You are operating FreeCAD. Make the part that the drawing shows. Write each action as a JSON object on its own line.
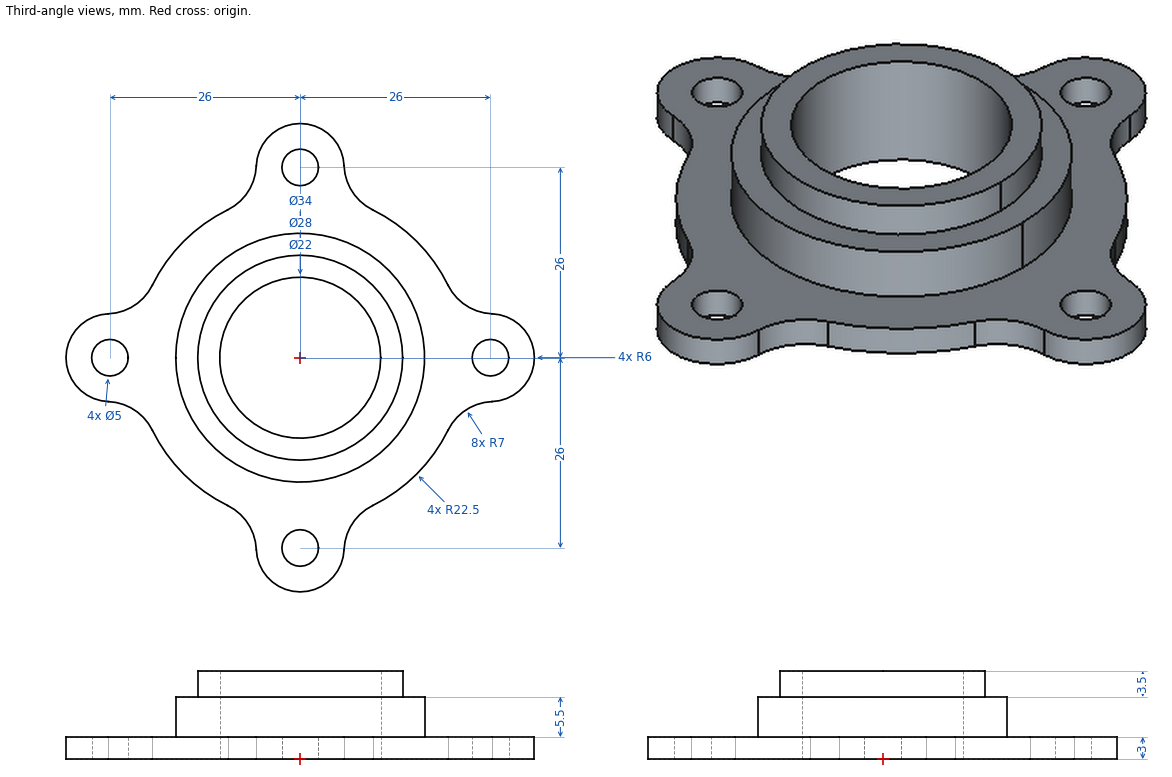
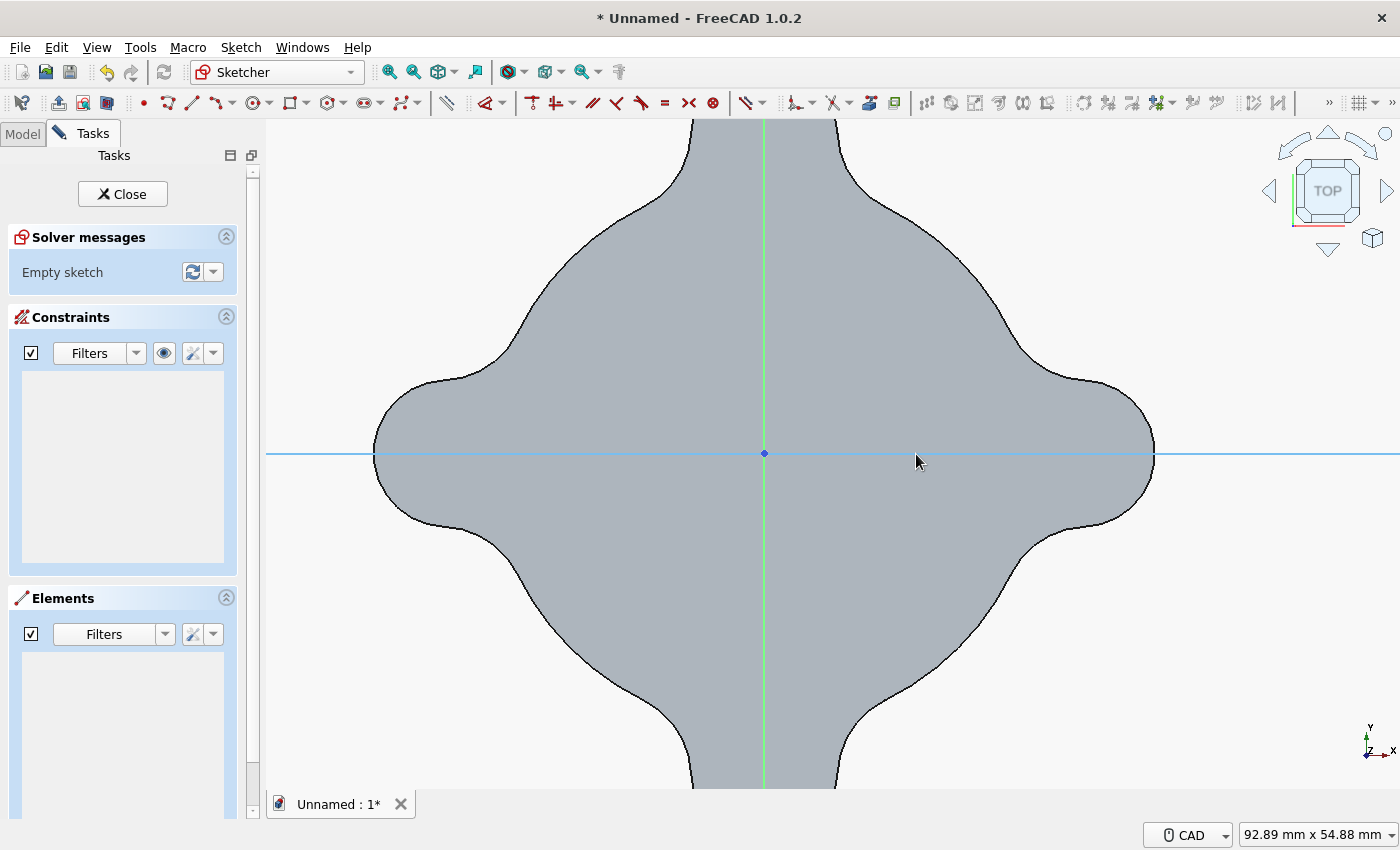
{"action": "left_click", "coordinate": [254, 104]}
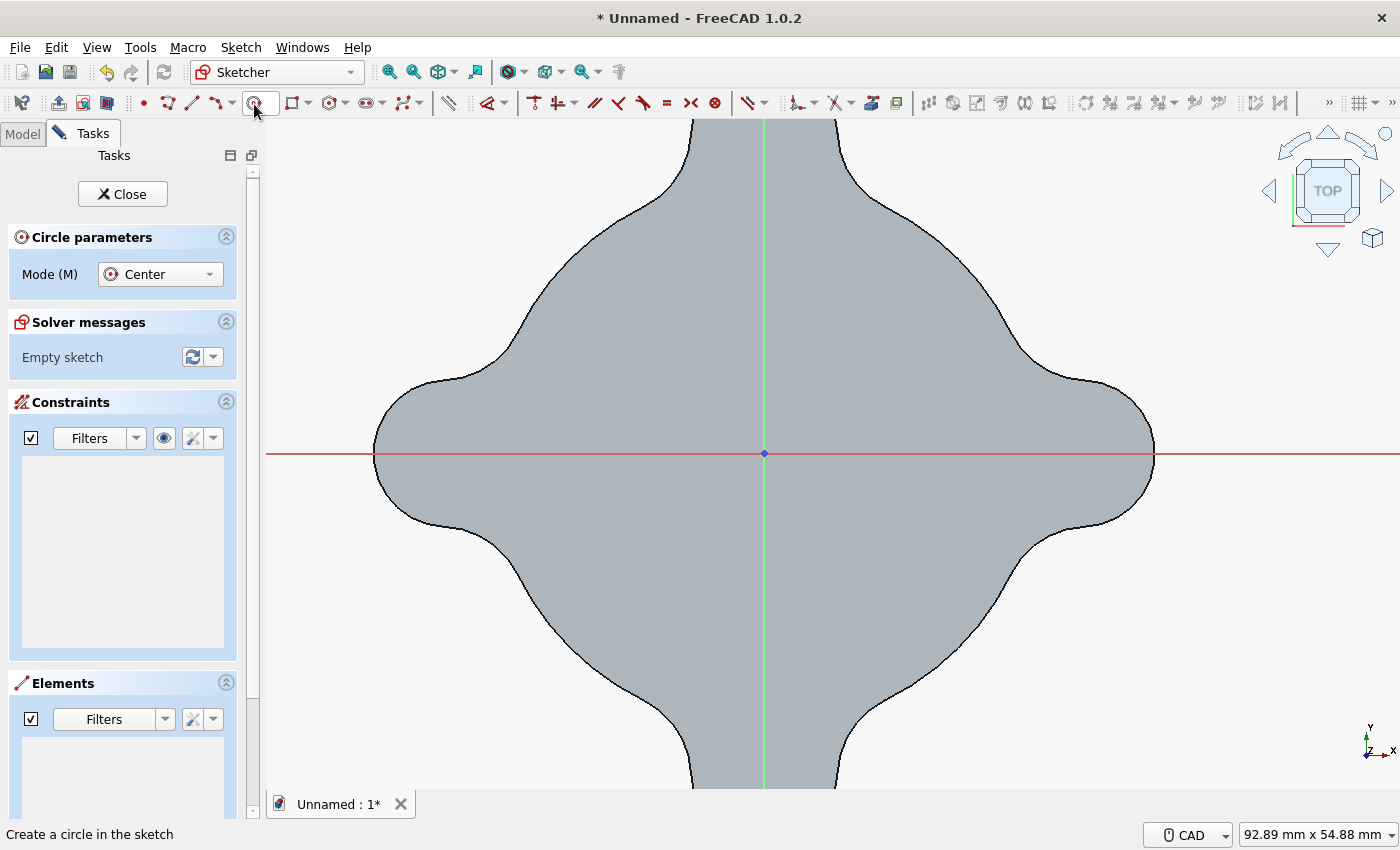
{"action": "left_click", "coordinate": [764, 454]}
{"action": "mouse_move", "coordinate": [911, 307]}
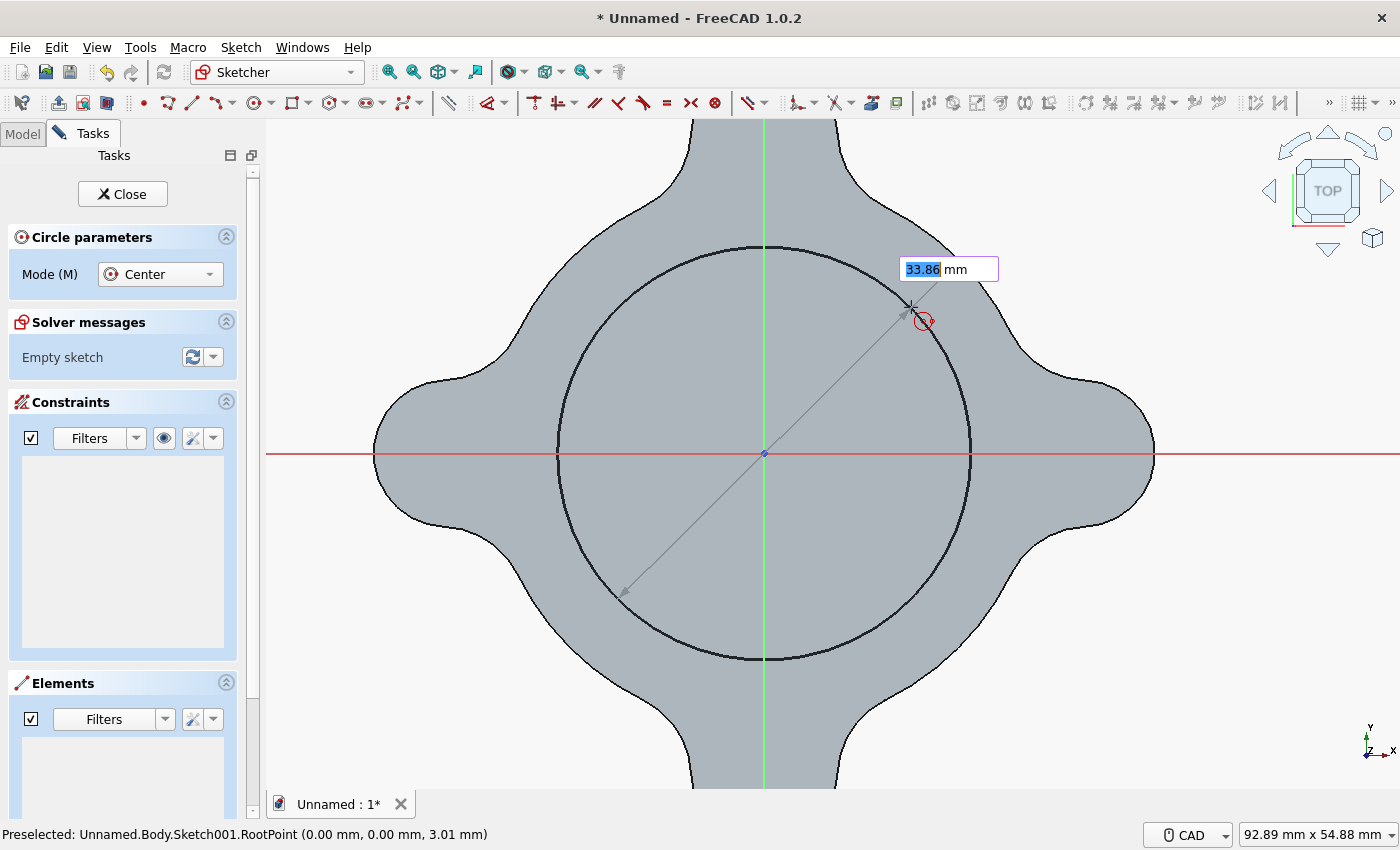
{"action": "type", "text": "34"}
{"action": "key", "text": "Return"}
{"action": "key", "text": "Escape"}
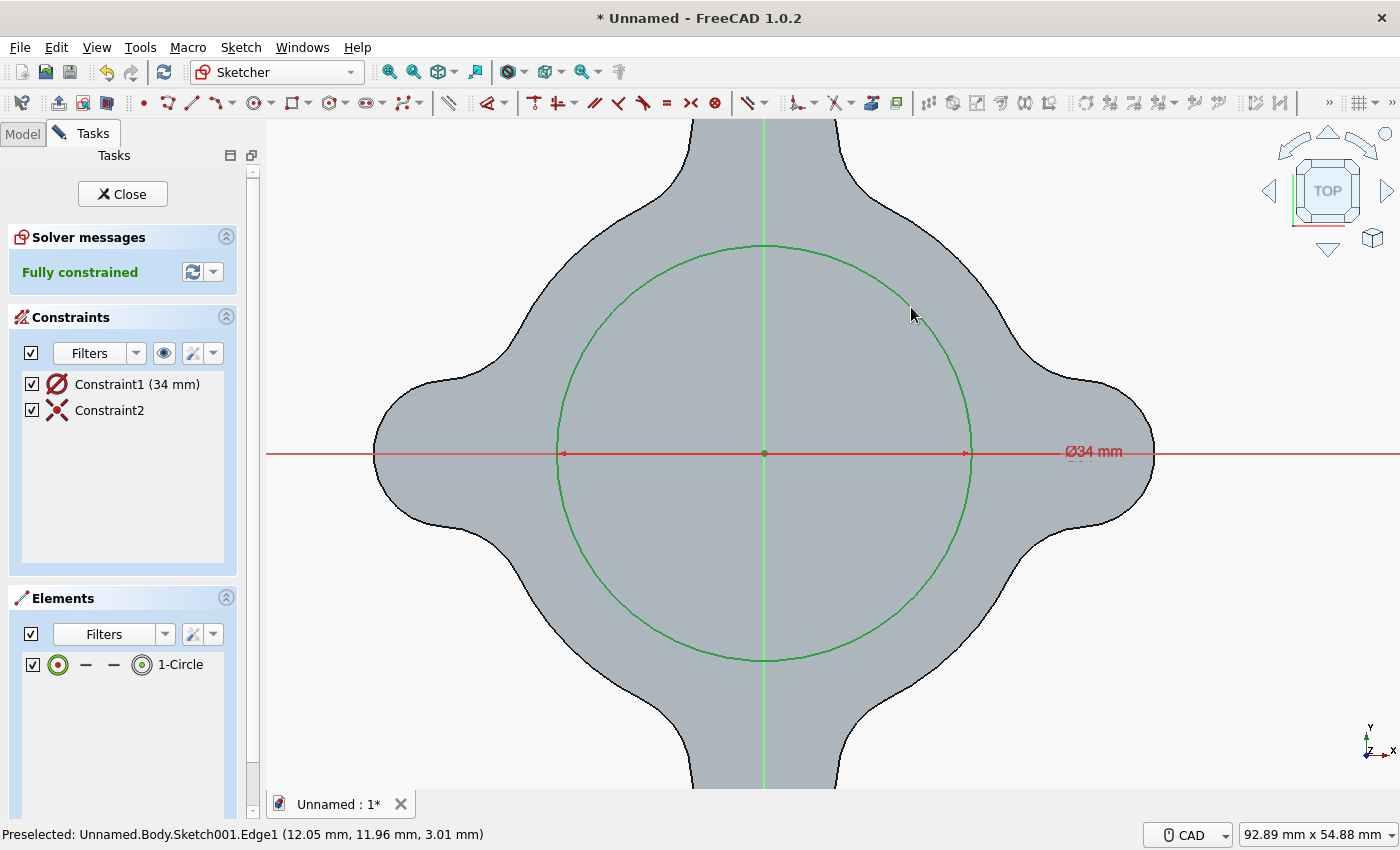
{"action": "left_click", "coordinate": [123, 194]}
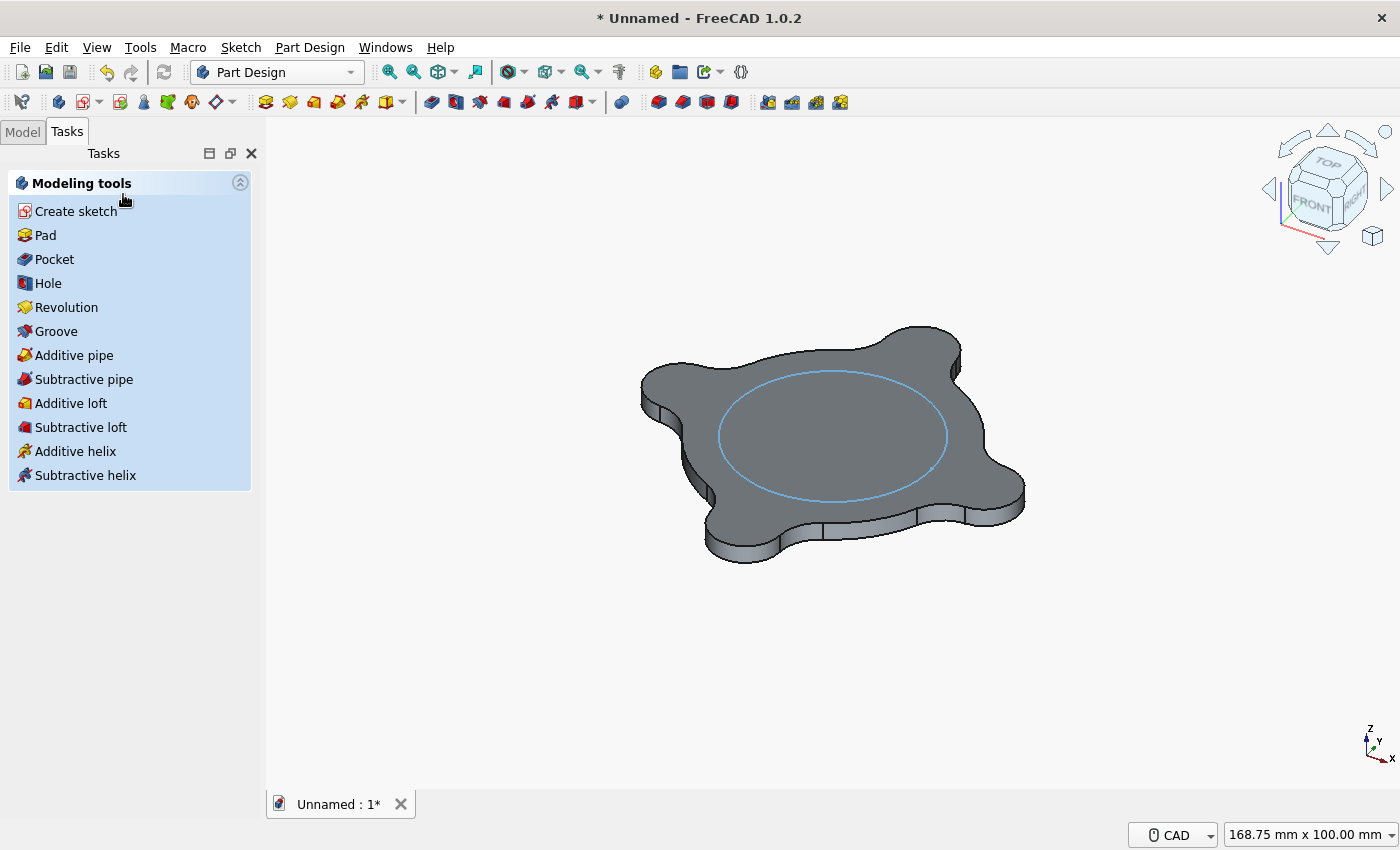
{"action": "left_click", "coordinate": [266, 102]}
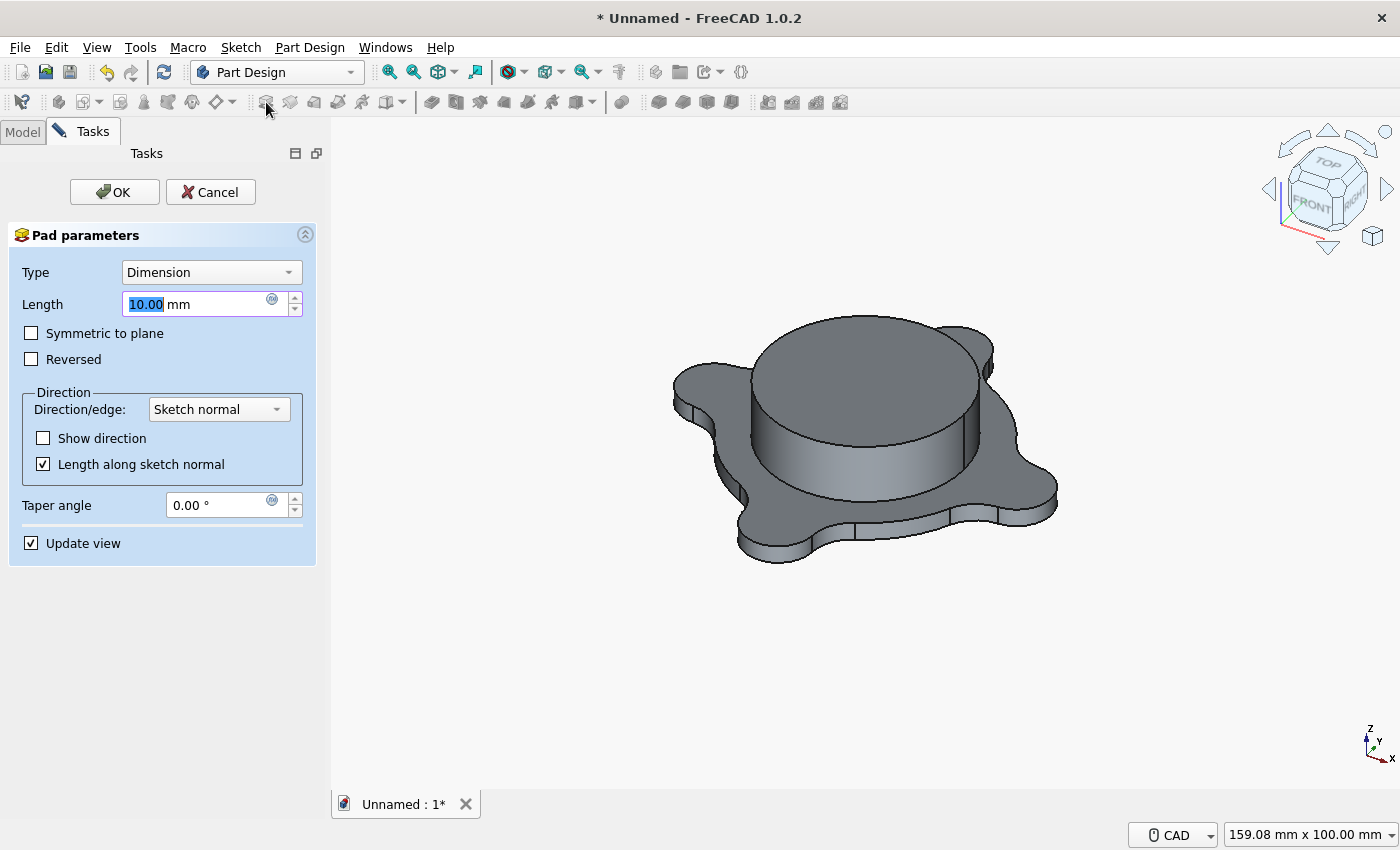
{"action": "type", "text": "5.5"}
{"action": "key", "text": "Tab"}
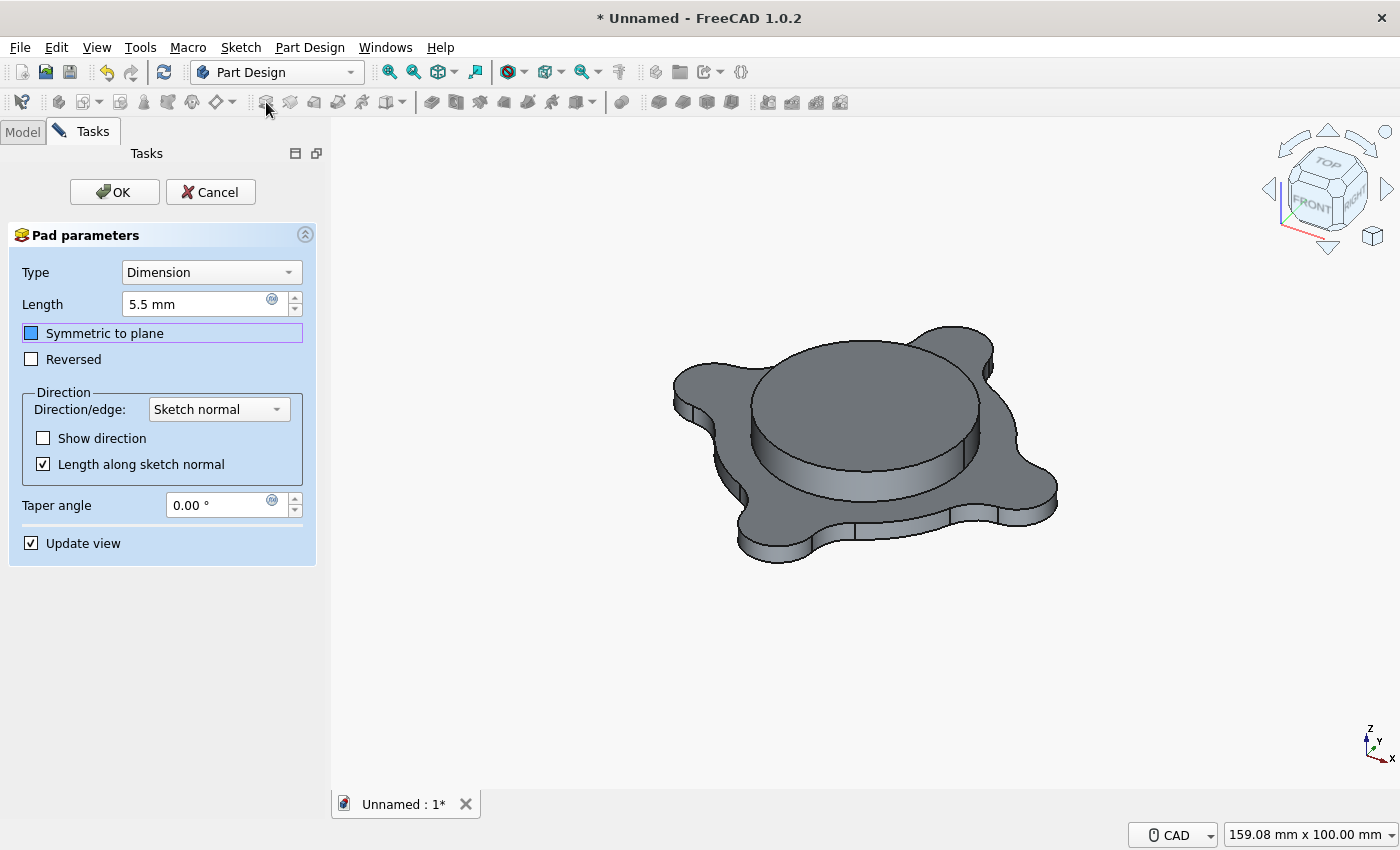
{"action": "left_click", "coordinate": [115, 192]}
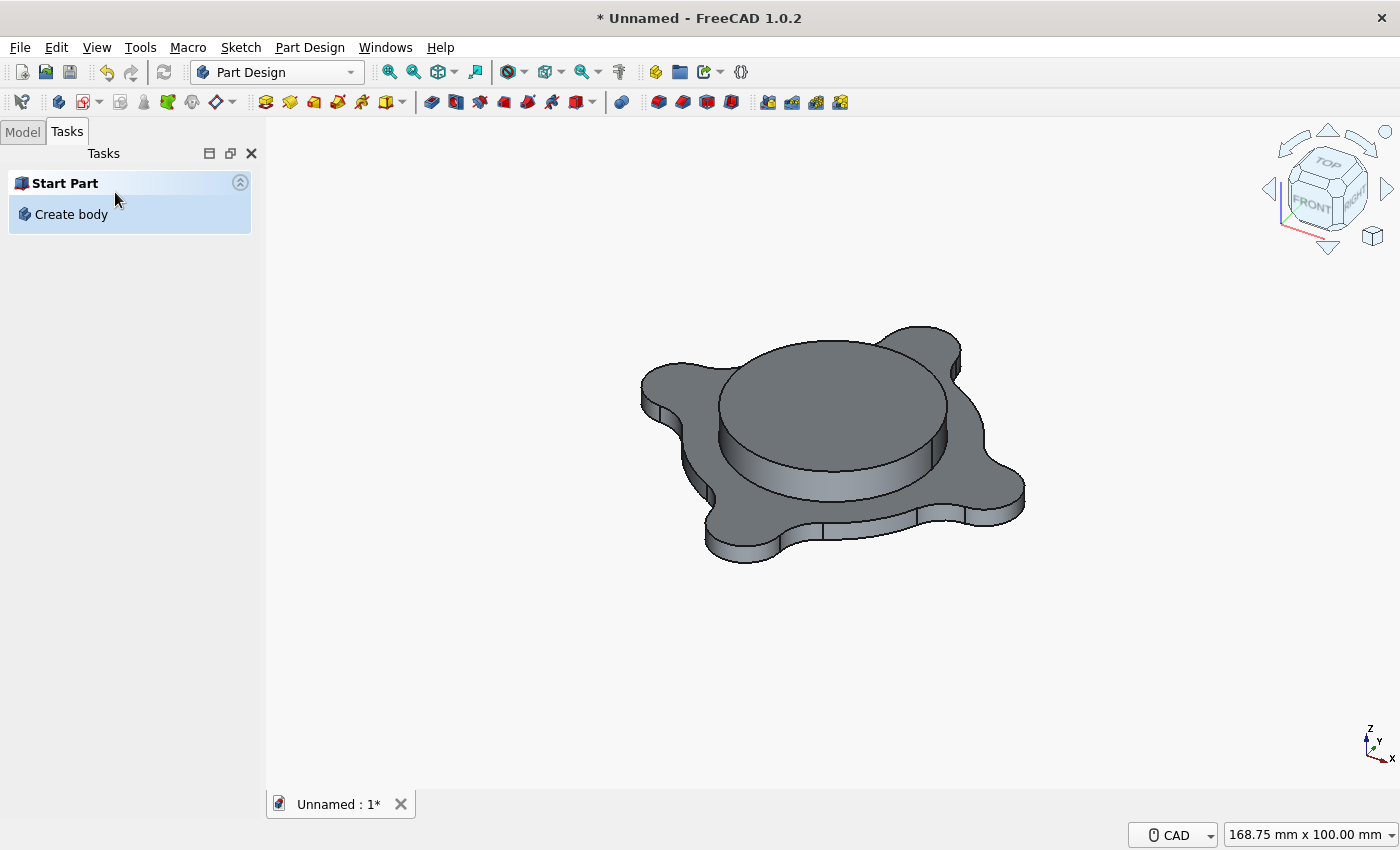
{"action": "left_click", "coordinate": [833, 405]}